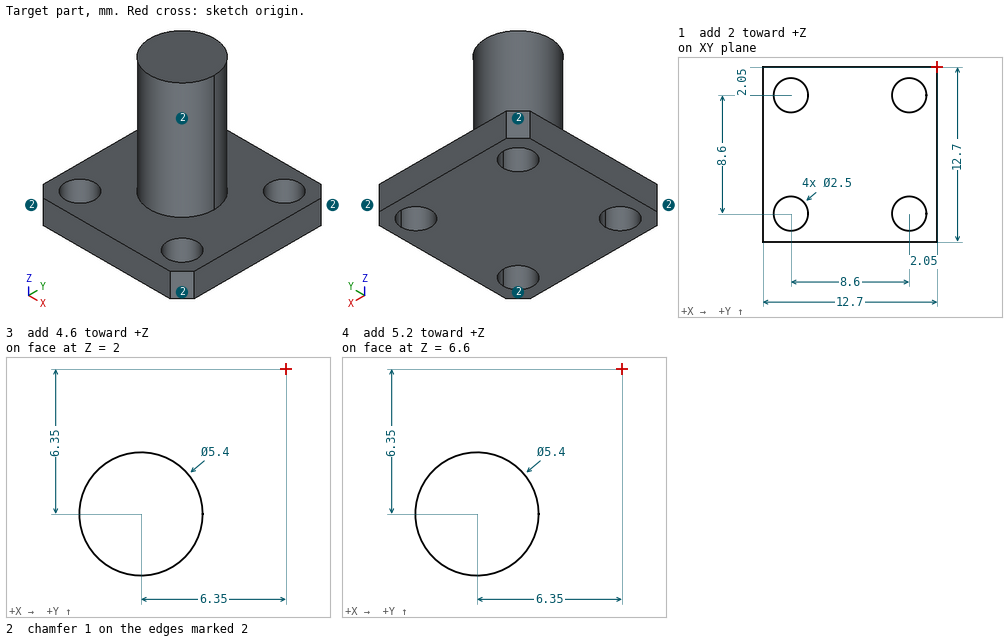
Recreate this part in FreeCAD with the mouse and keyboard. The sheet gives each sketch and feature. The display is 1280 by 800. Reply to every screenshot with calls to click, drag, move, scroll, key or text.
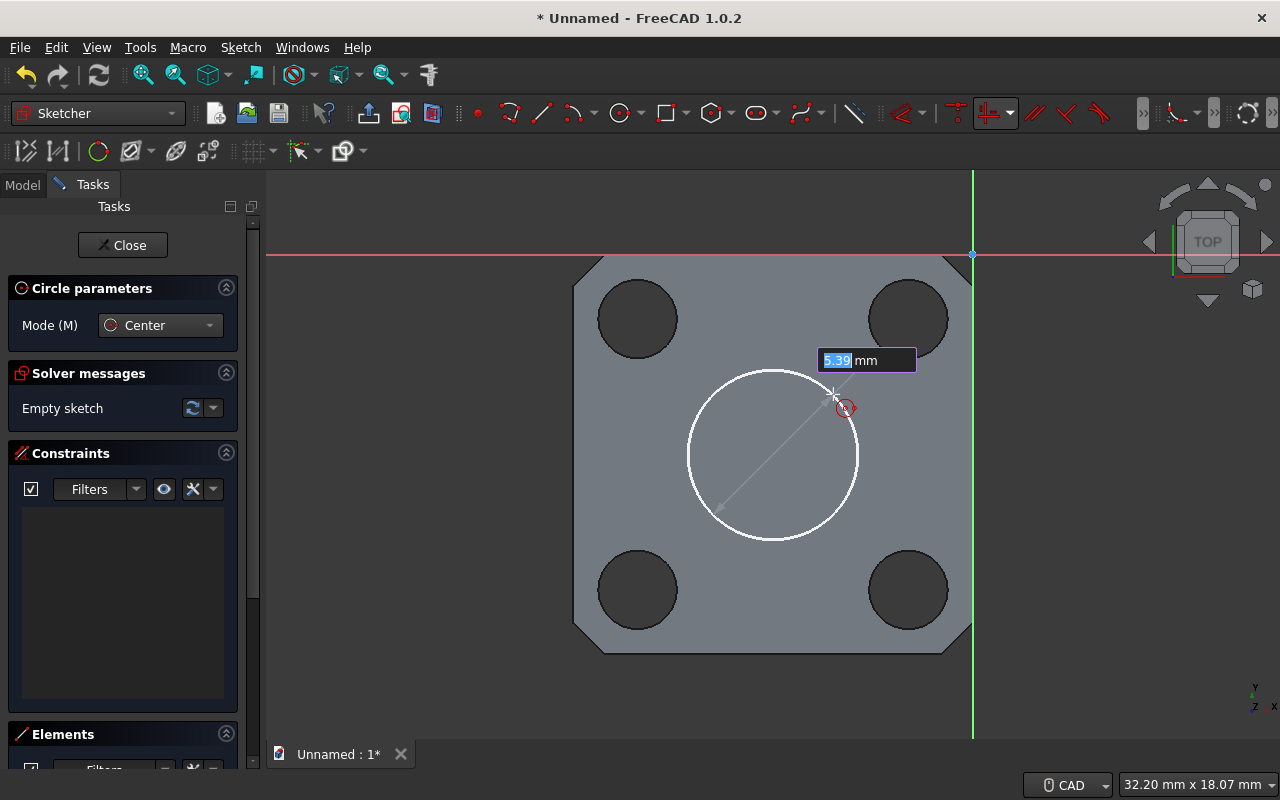
text(5.4)
key(Return)
key(Escape)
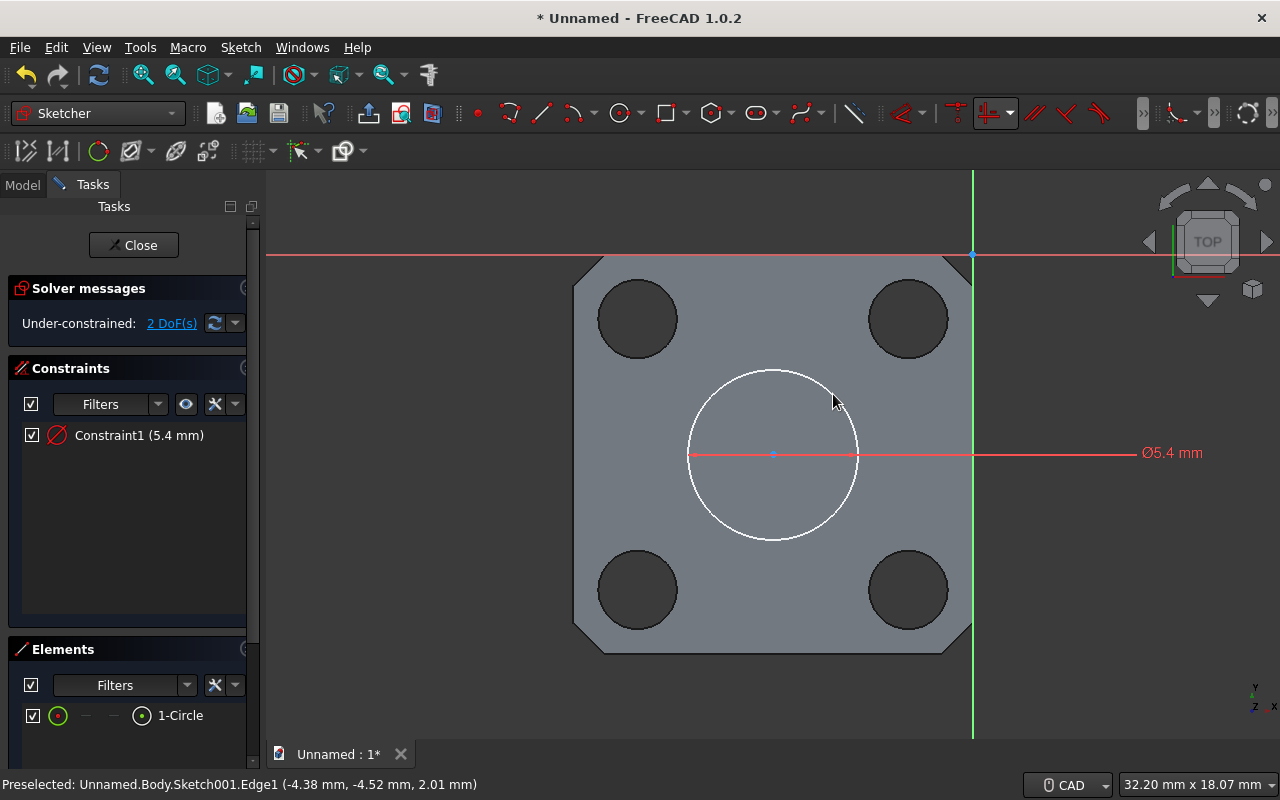
click(902, 114)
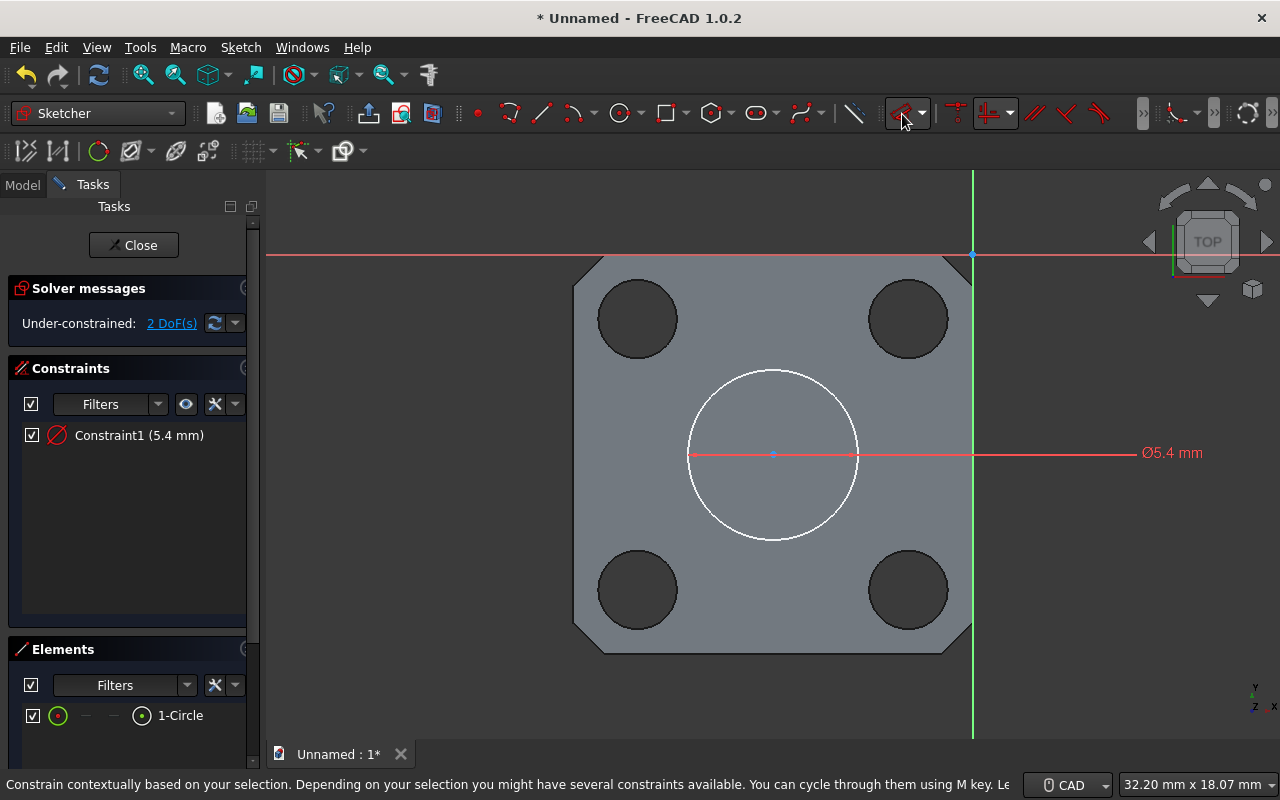
click(773, 455)
click(873, 221)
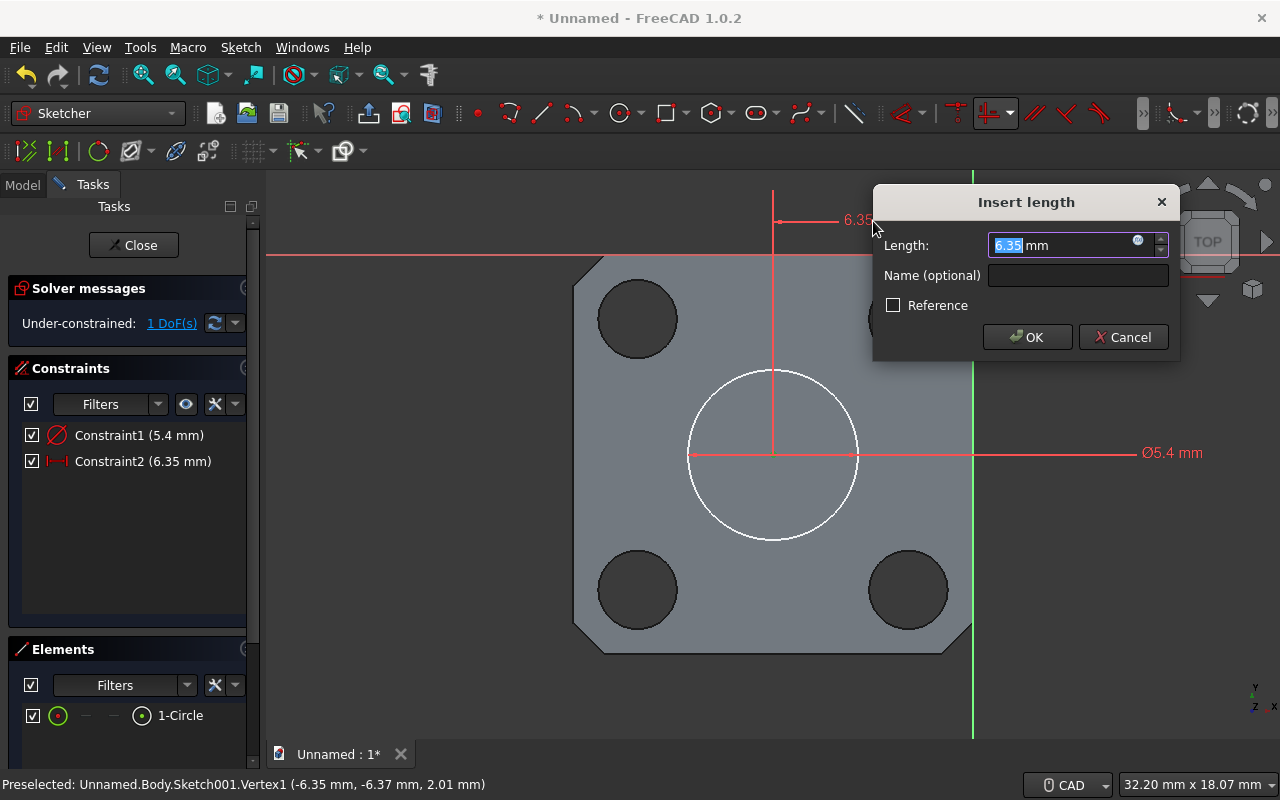
text(6.35)
key(Return)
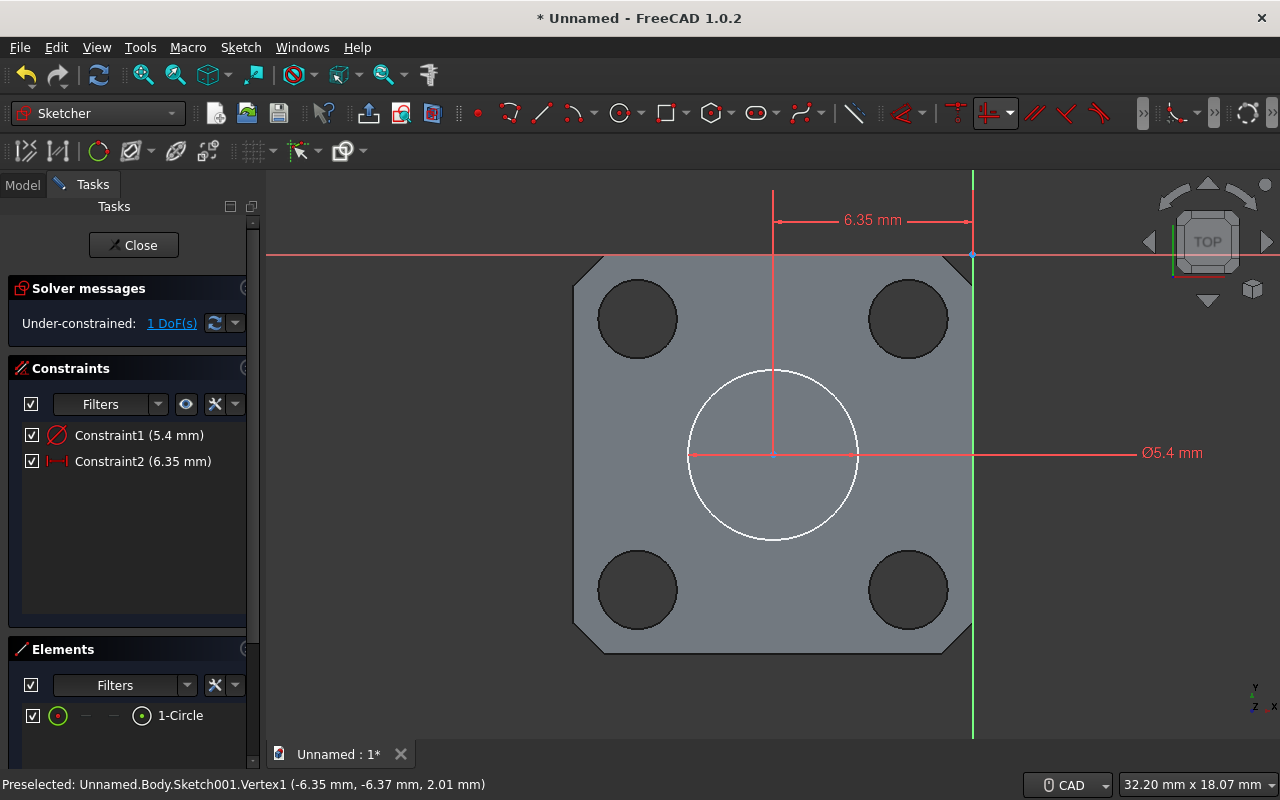
click(773, 455)
click(1007, 355)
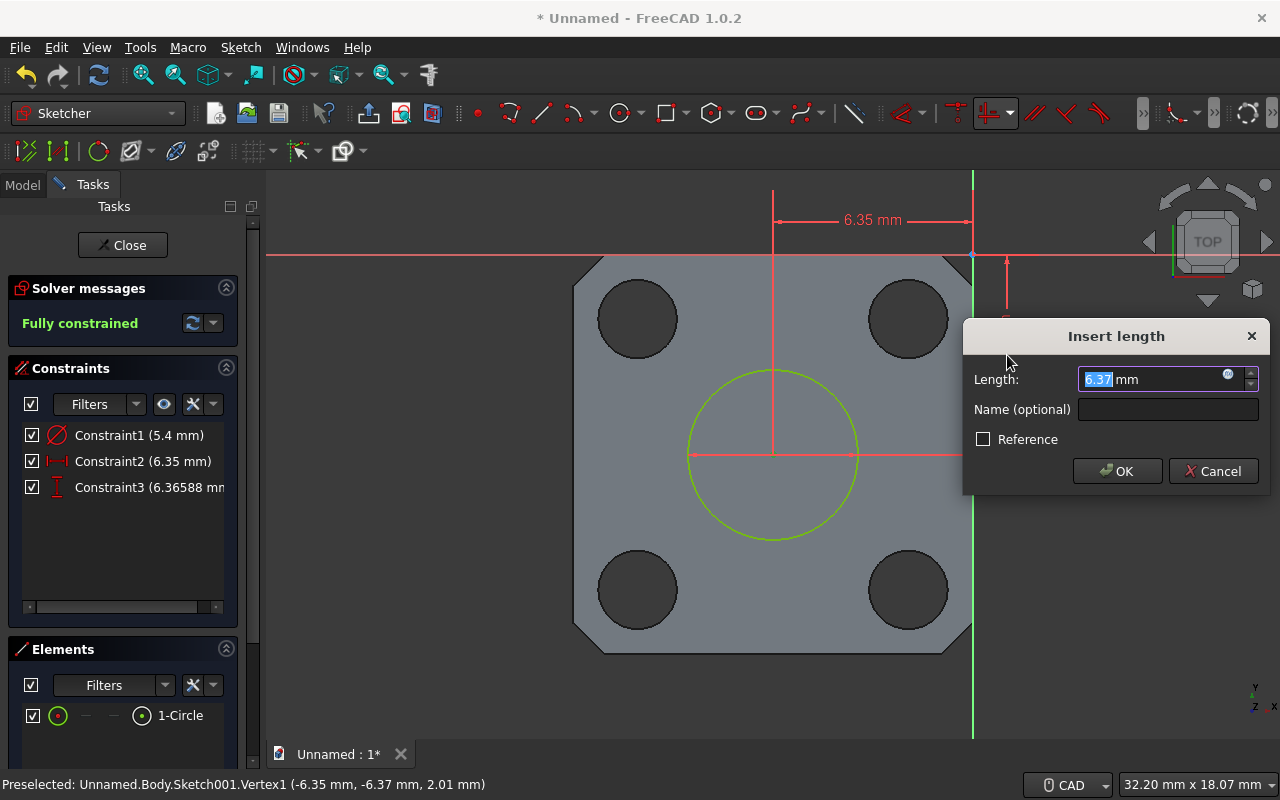
text(6.35)
key(Return)
key(Escape)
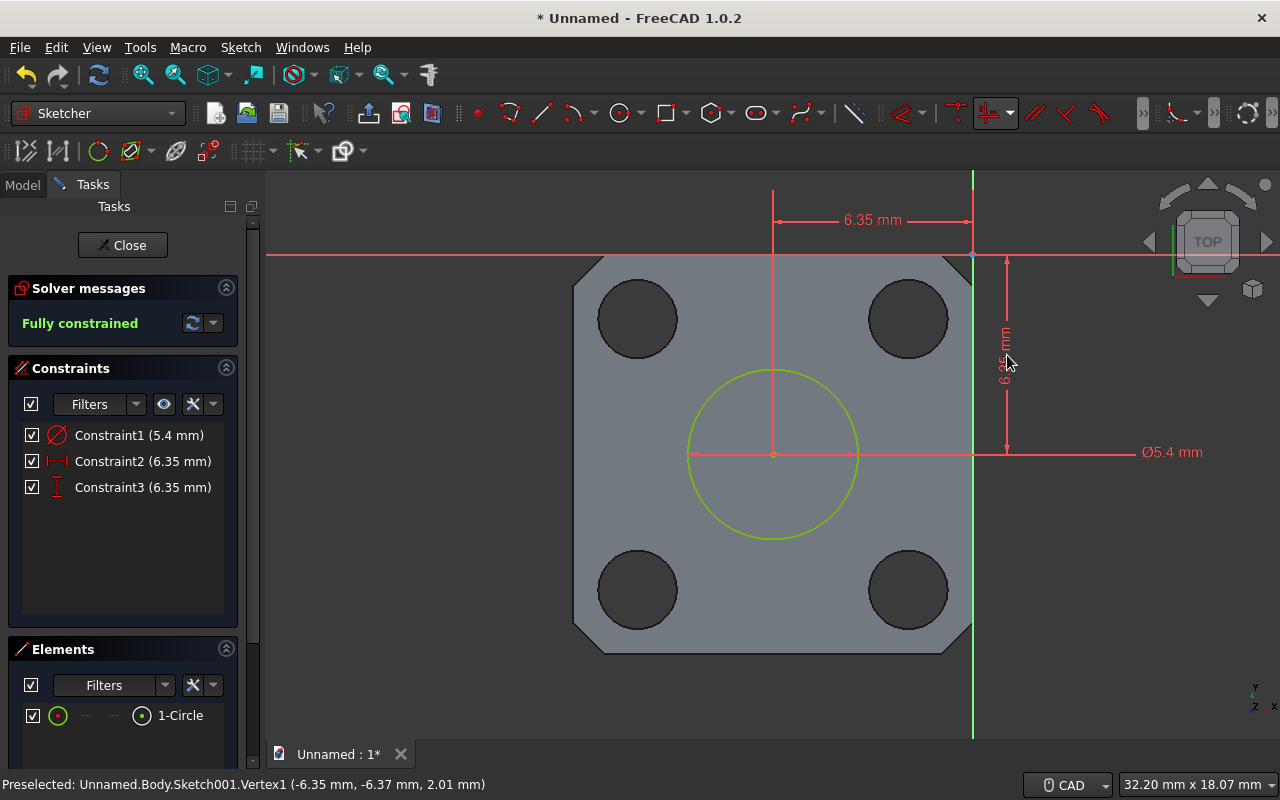
click(123, 245)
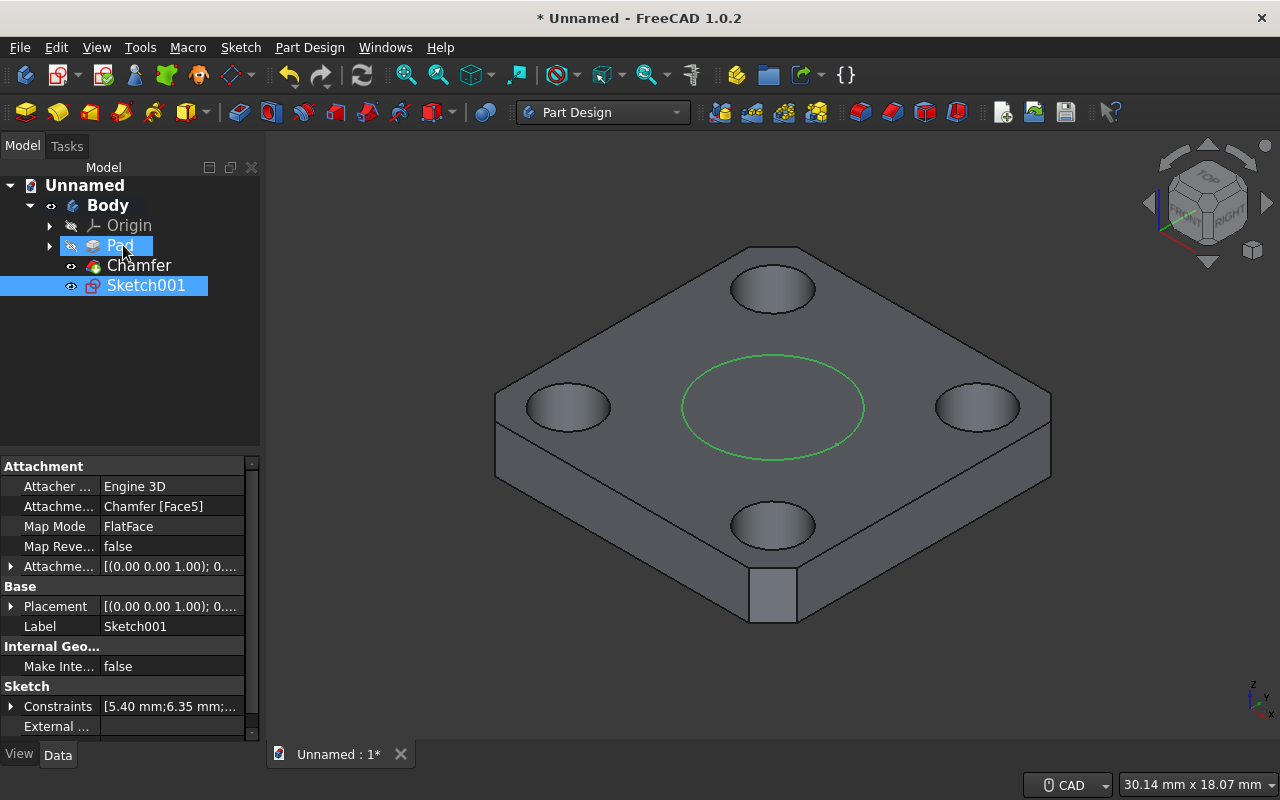
click(26, 112)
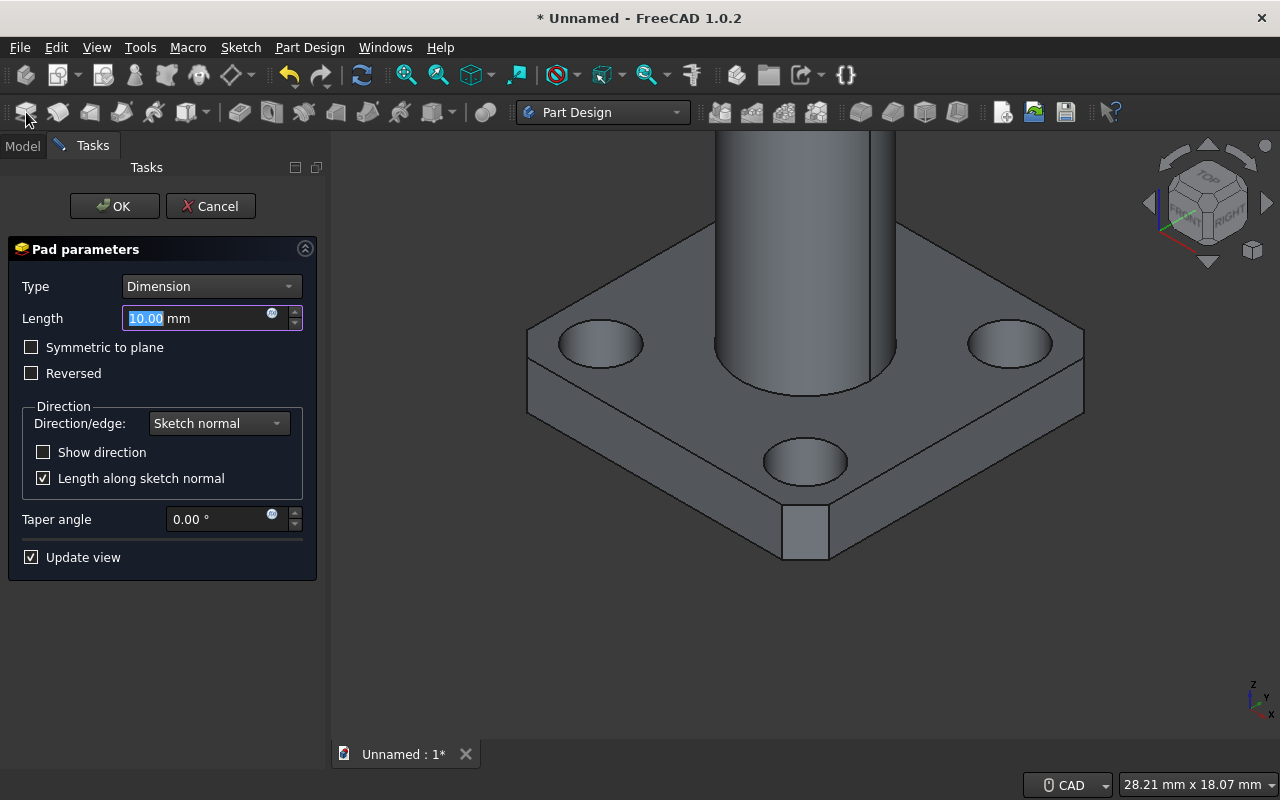
text(4.6)
key(Tab)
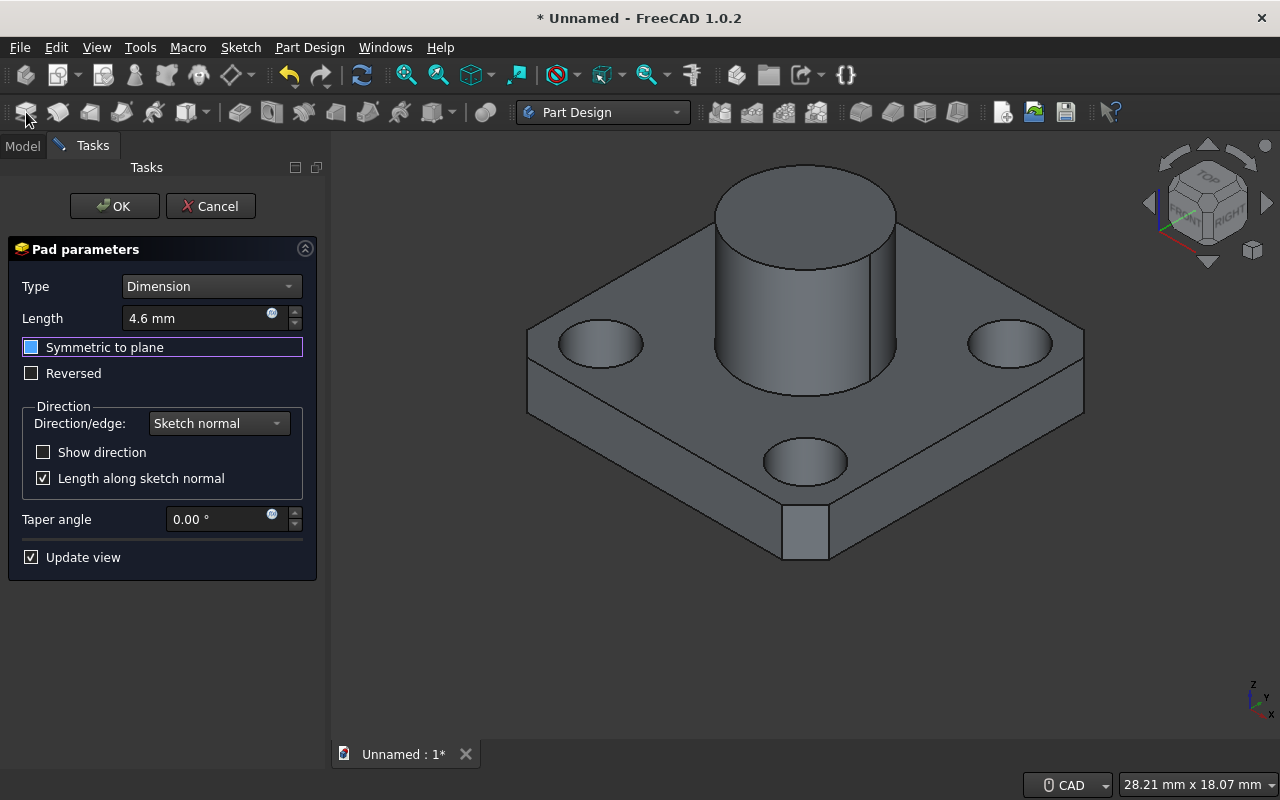
click(115, 206)